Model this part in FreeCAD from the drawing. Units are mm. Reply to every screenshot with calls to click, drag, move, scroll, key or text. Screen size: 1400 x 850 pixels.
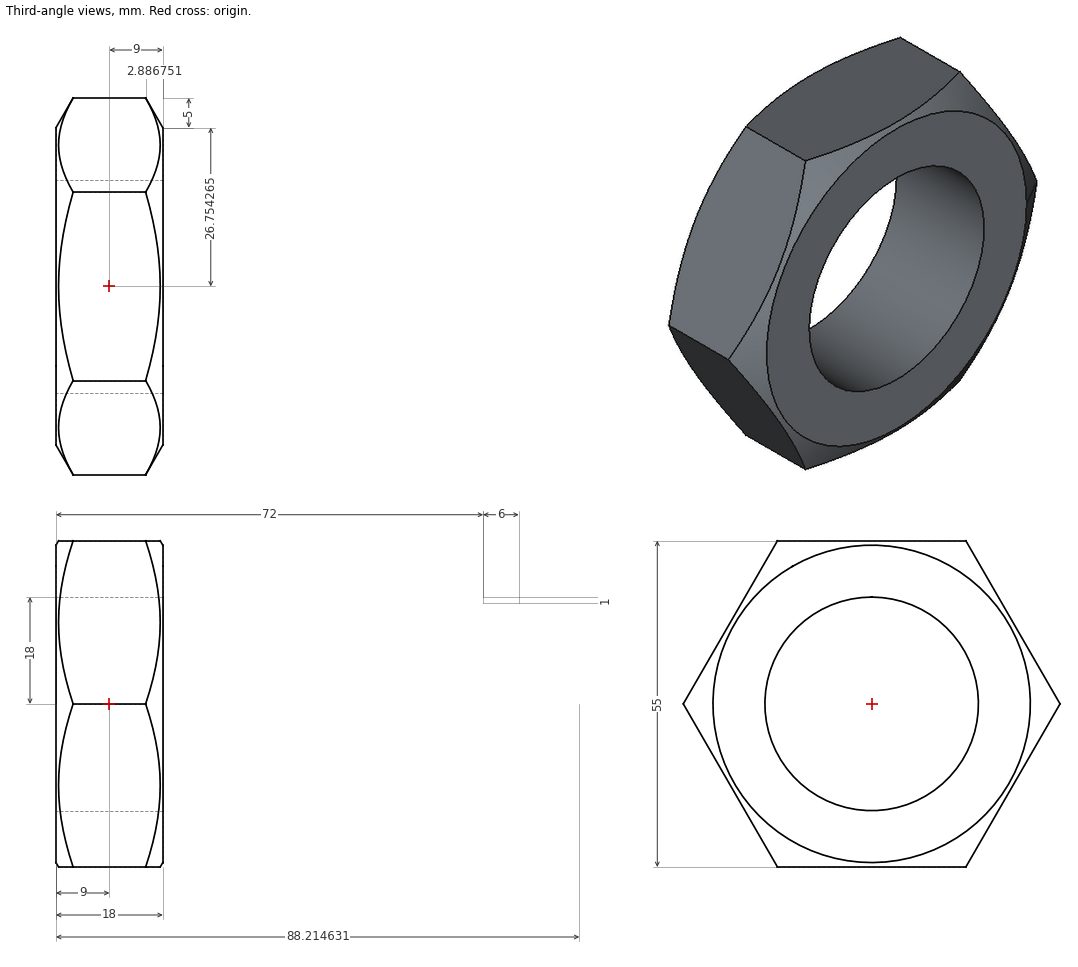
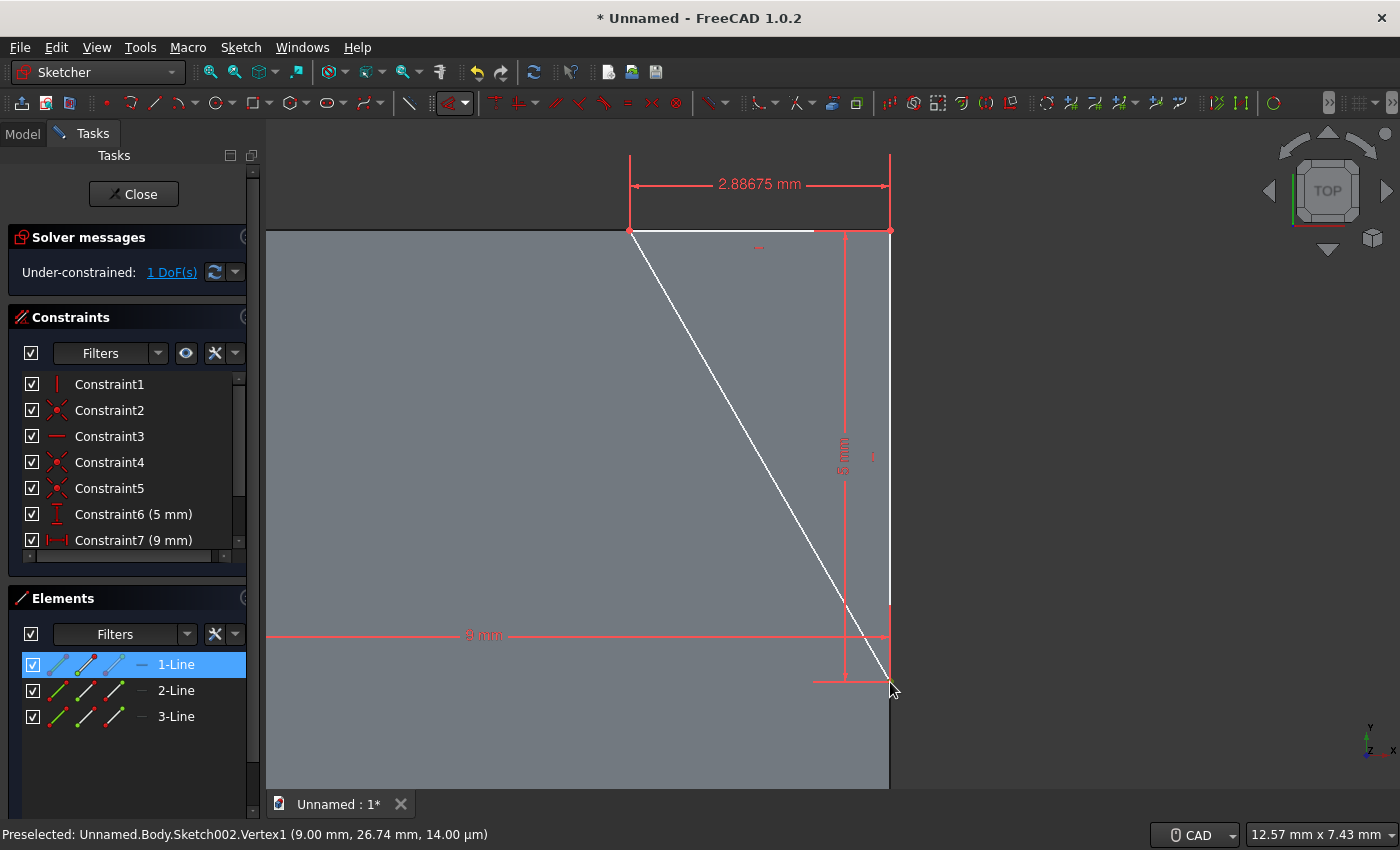
key(i)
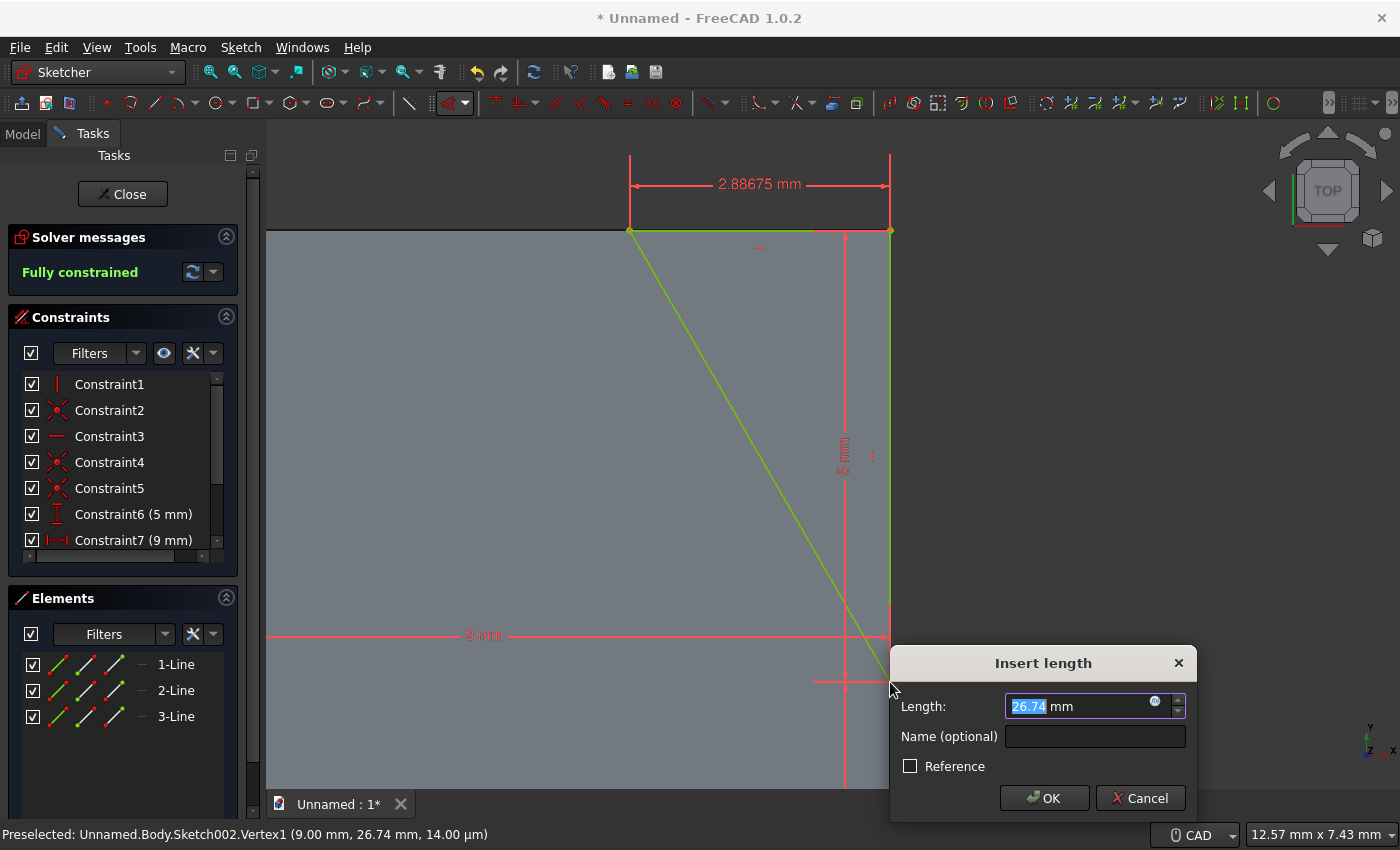
text(26.754265)
key(Return)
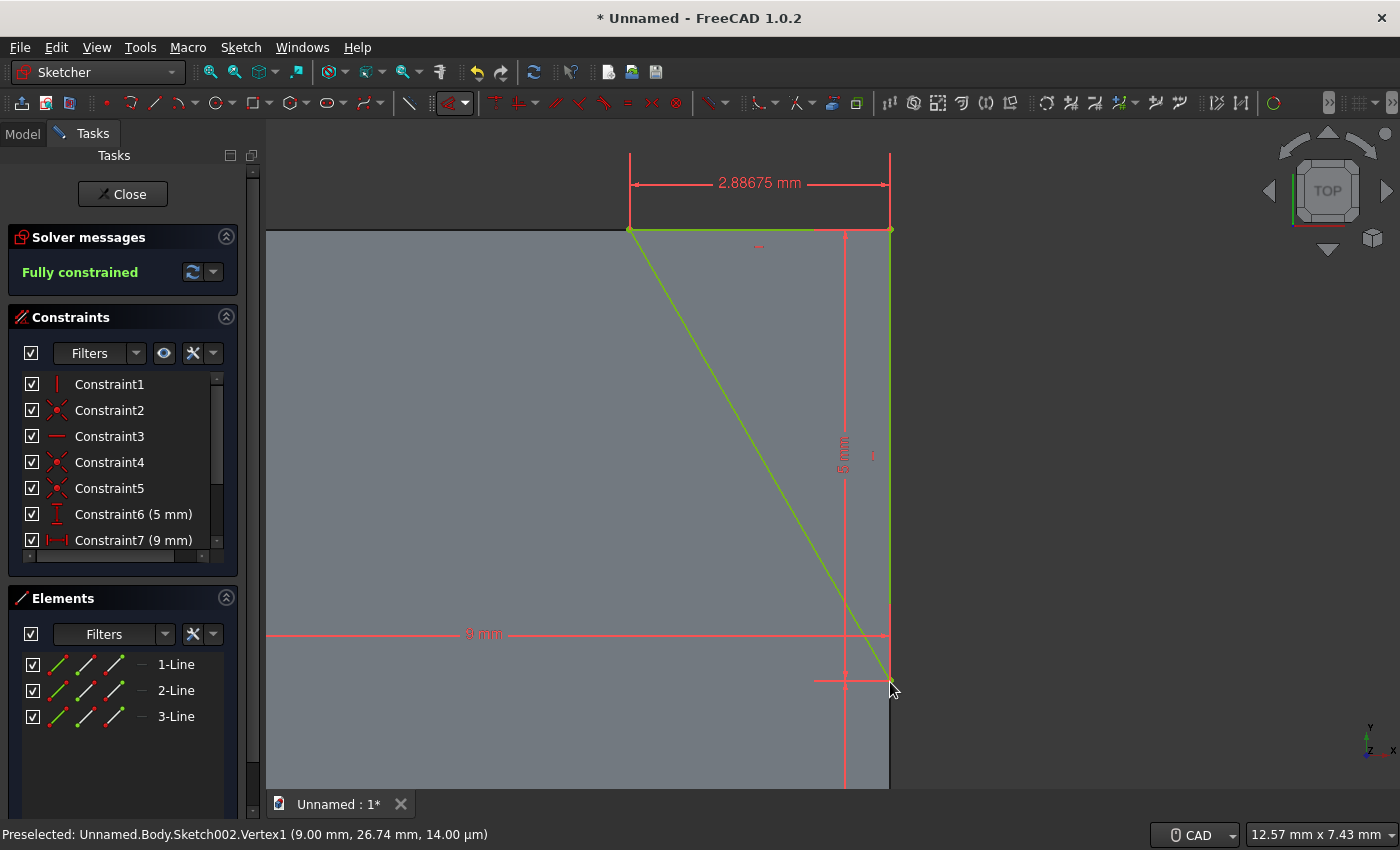
click(123, 194)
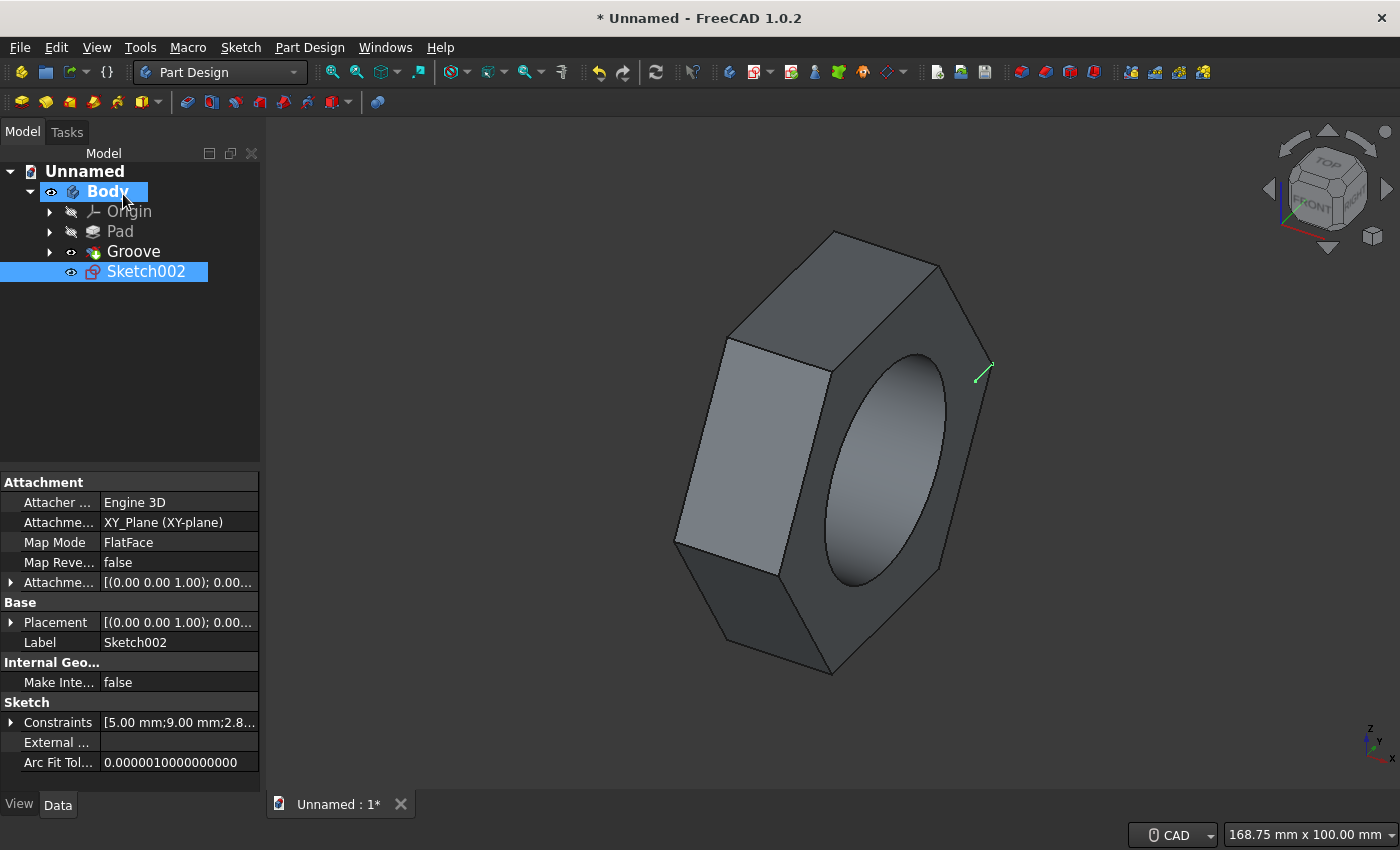
click(236, 102)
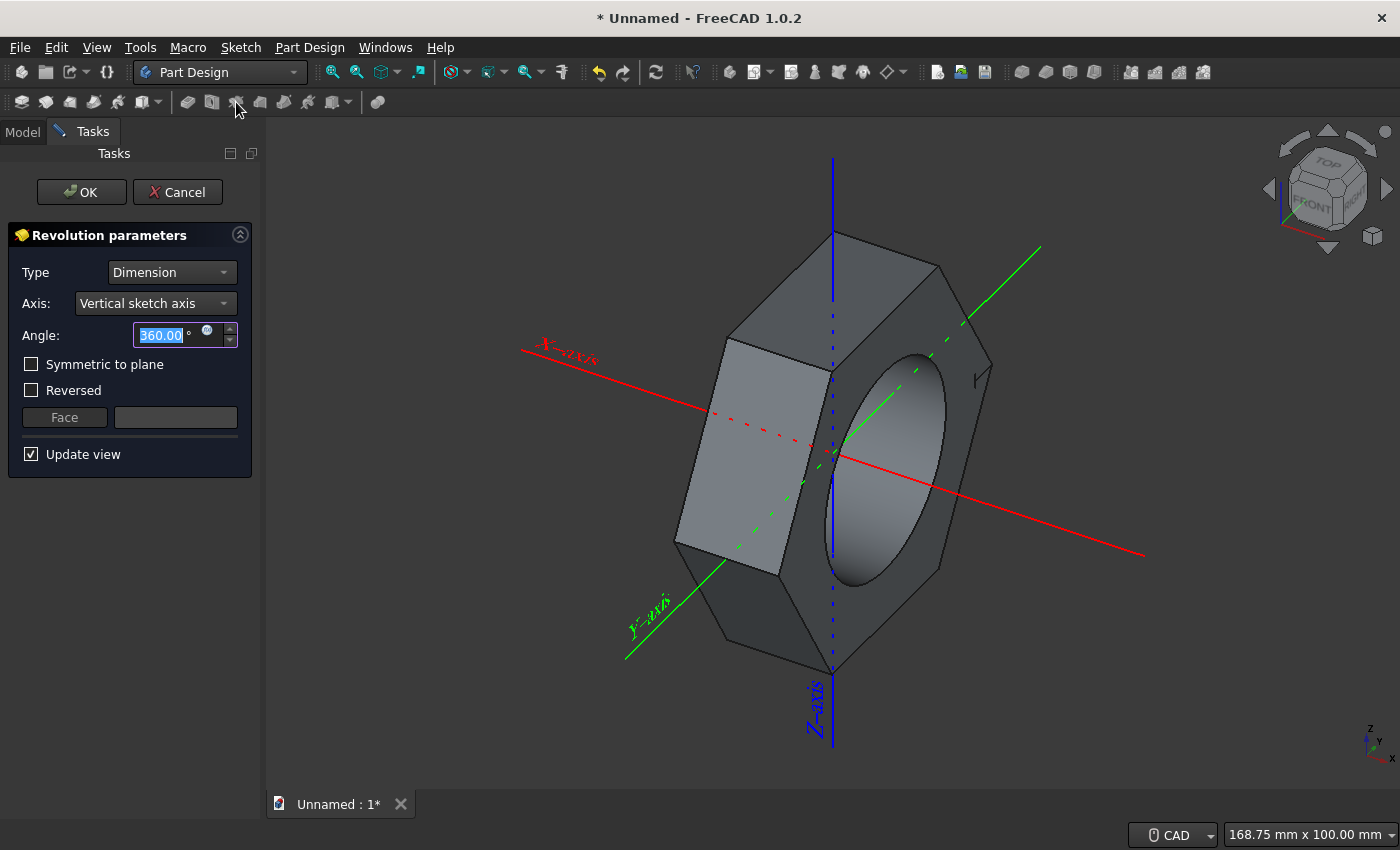
click(156, 304)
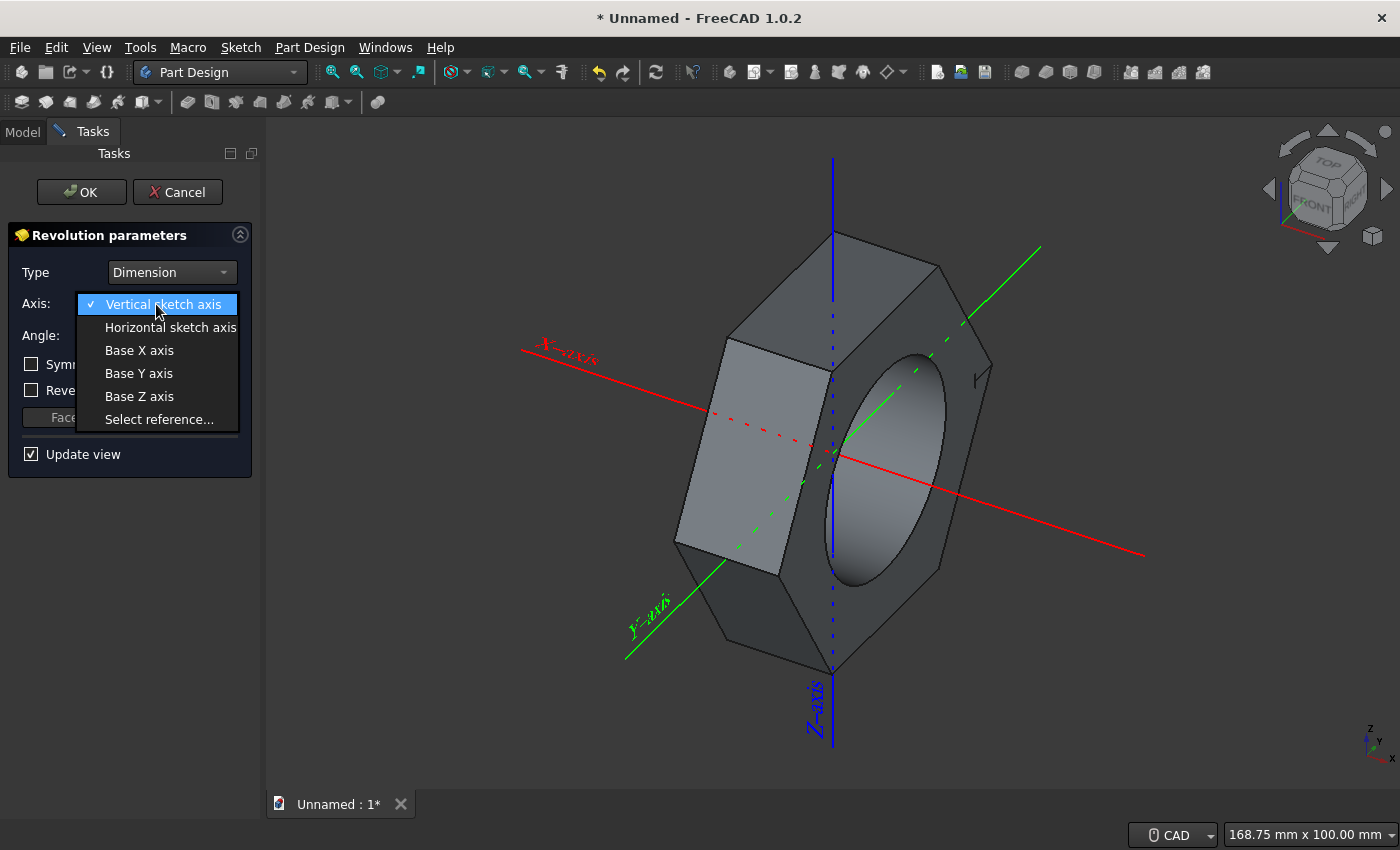
click(156, 328)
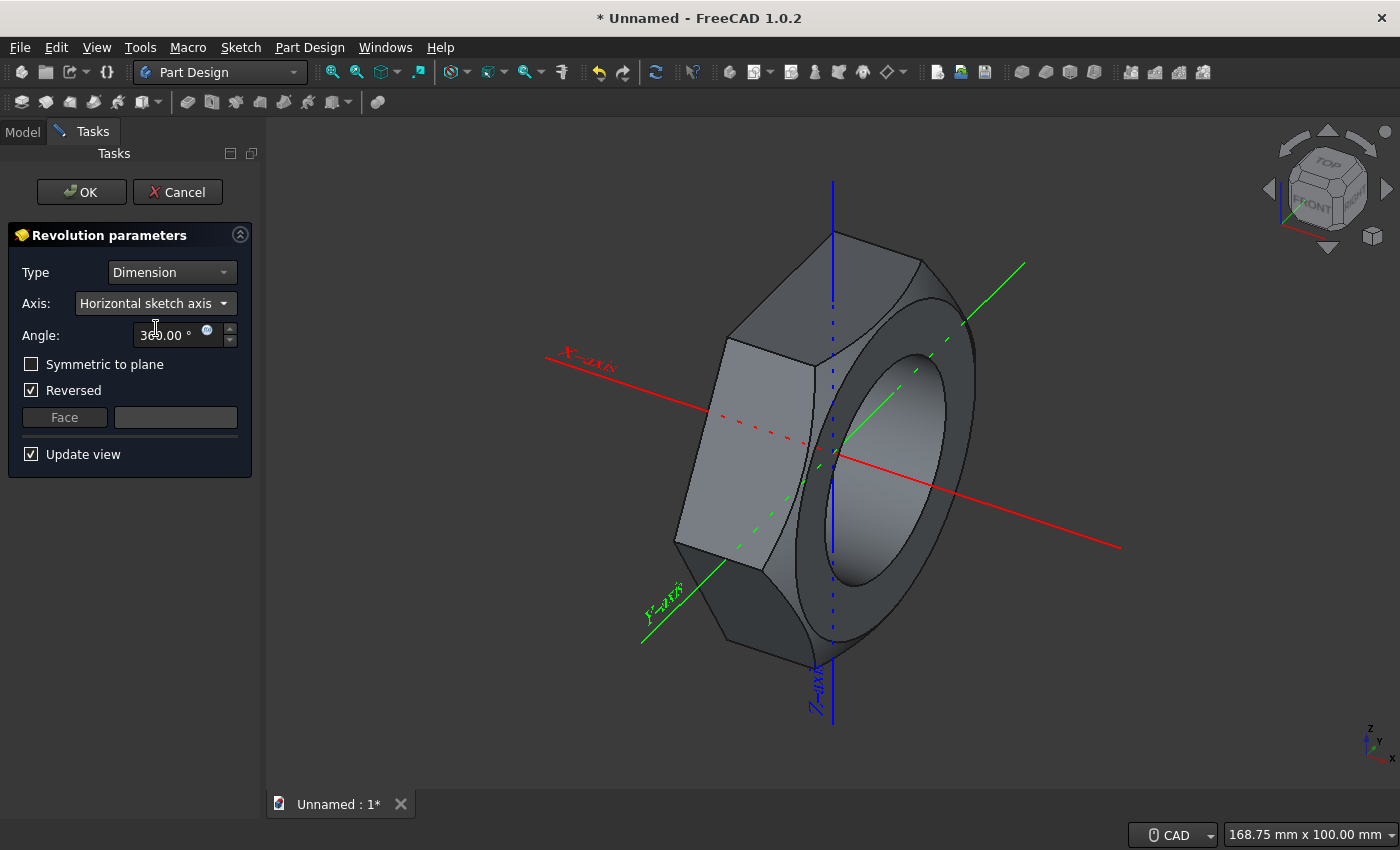
click(82, 192)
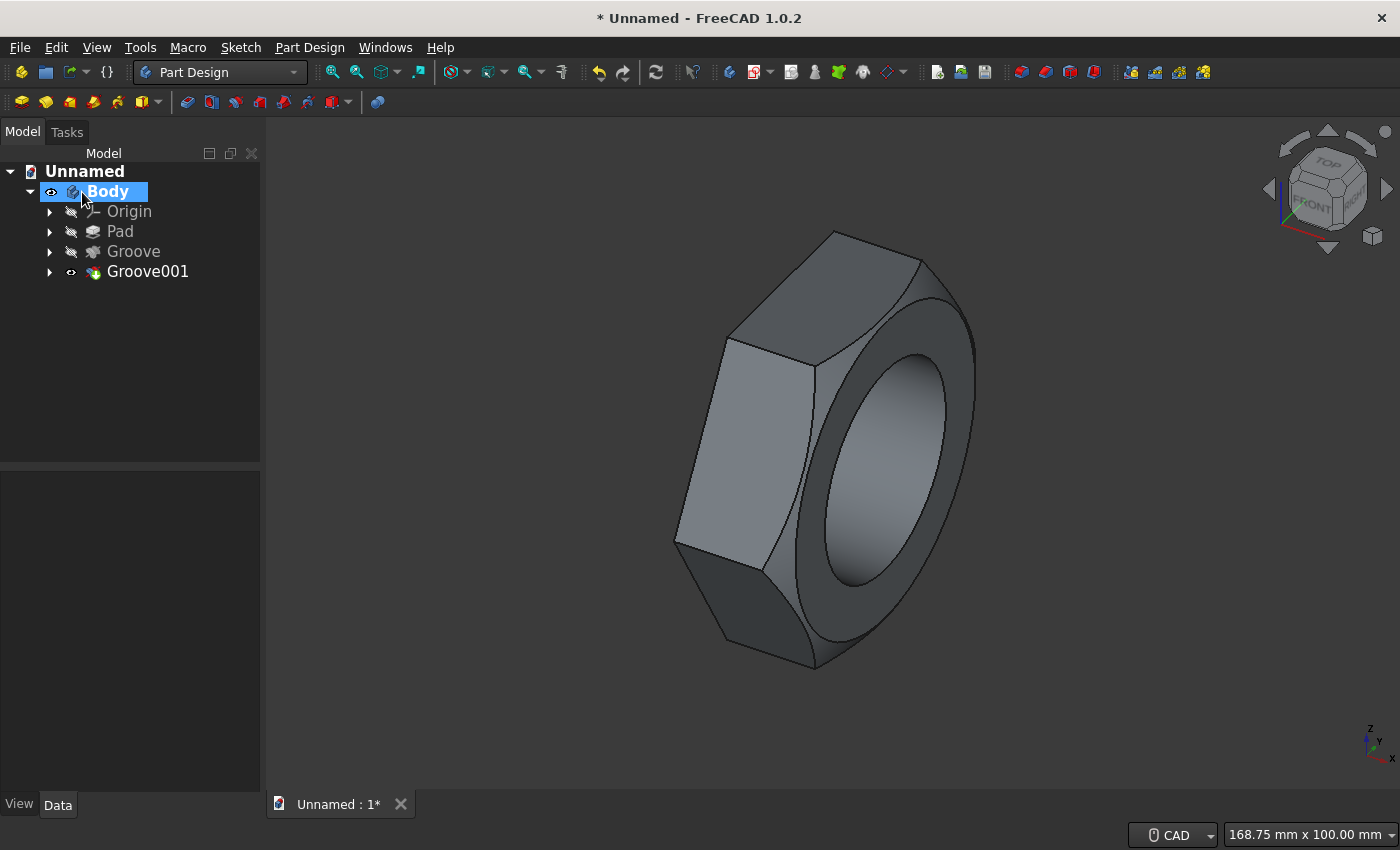
click(116, 272)